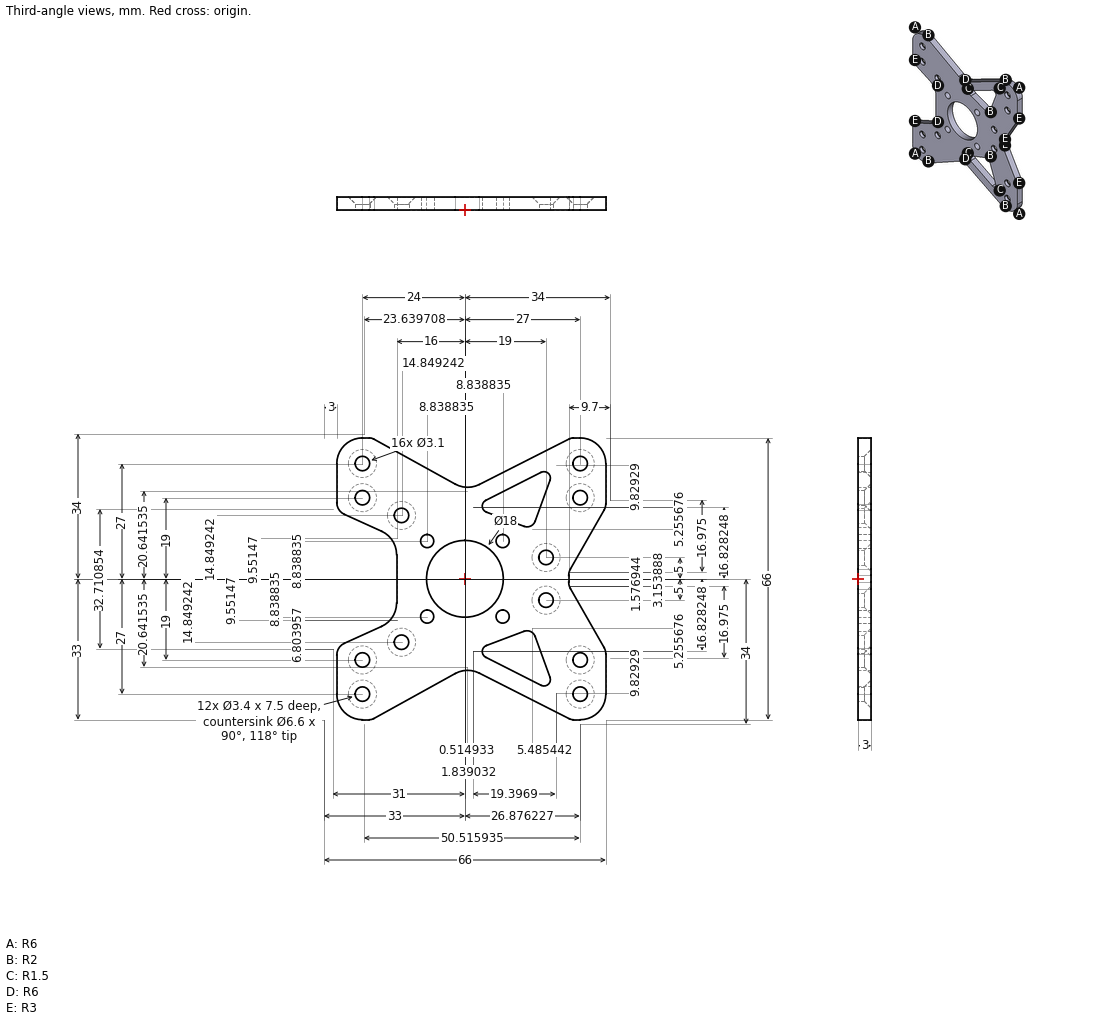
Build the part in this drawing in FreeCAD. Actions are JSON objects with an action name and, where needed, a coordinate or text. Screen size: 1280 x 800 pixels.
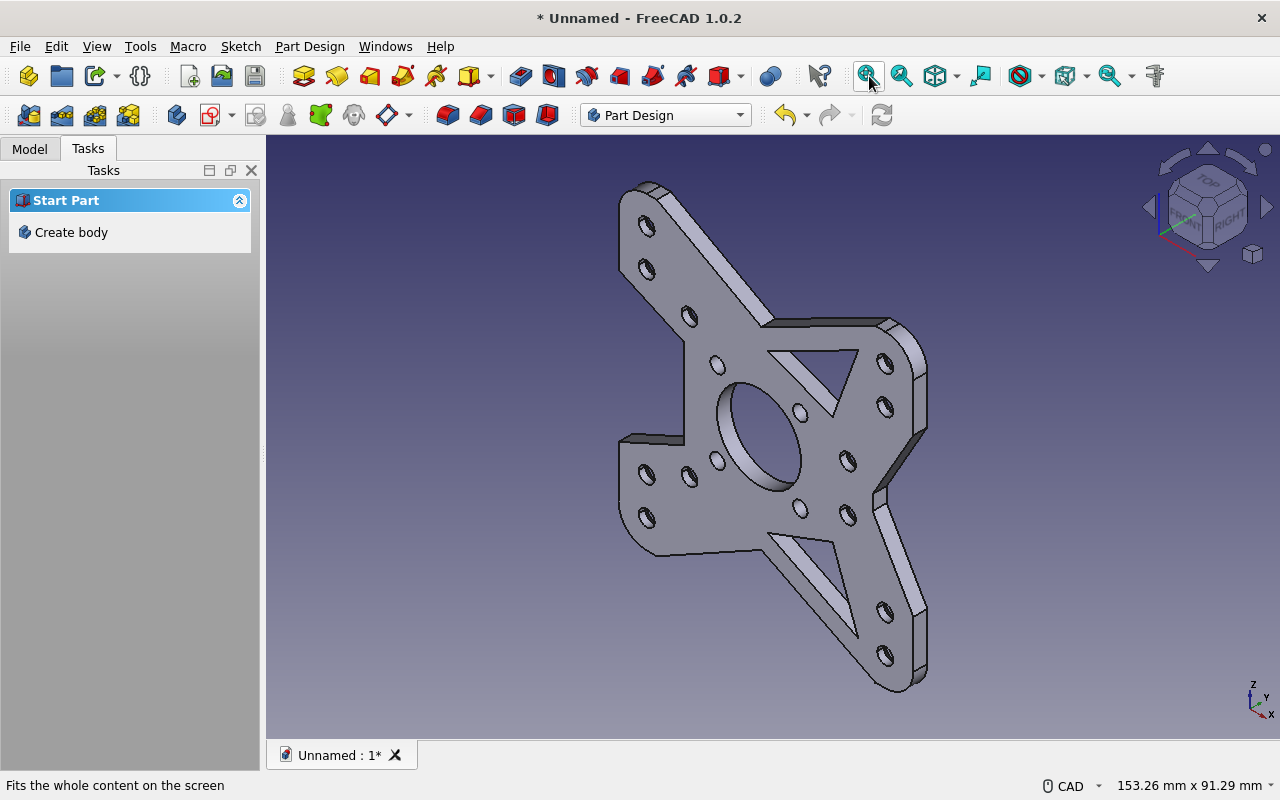
{"action": "key", "text": "2"}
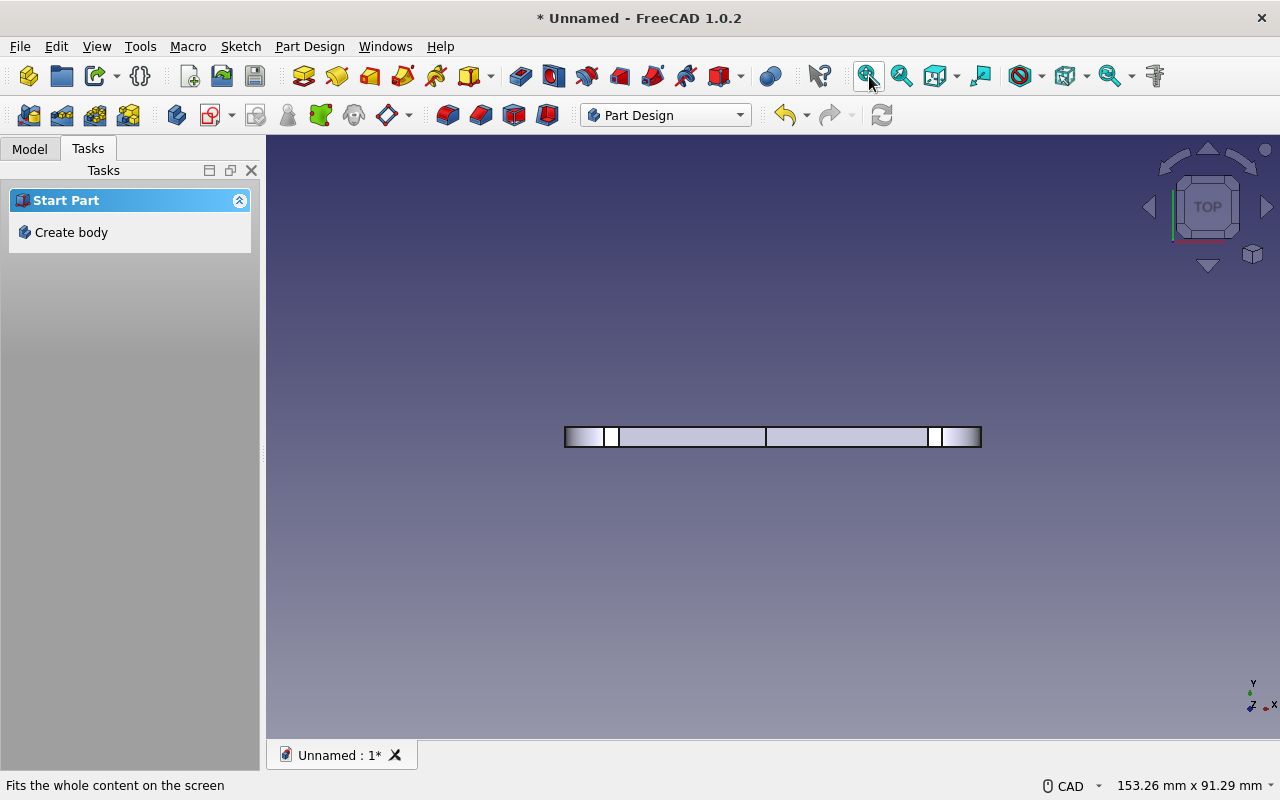
{"action": "key", "text": "v f"}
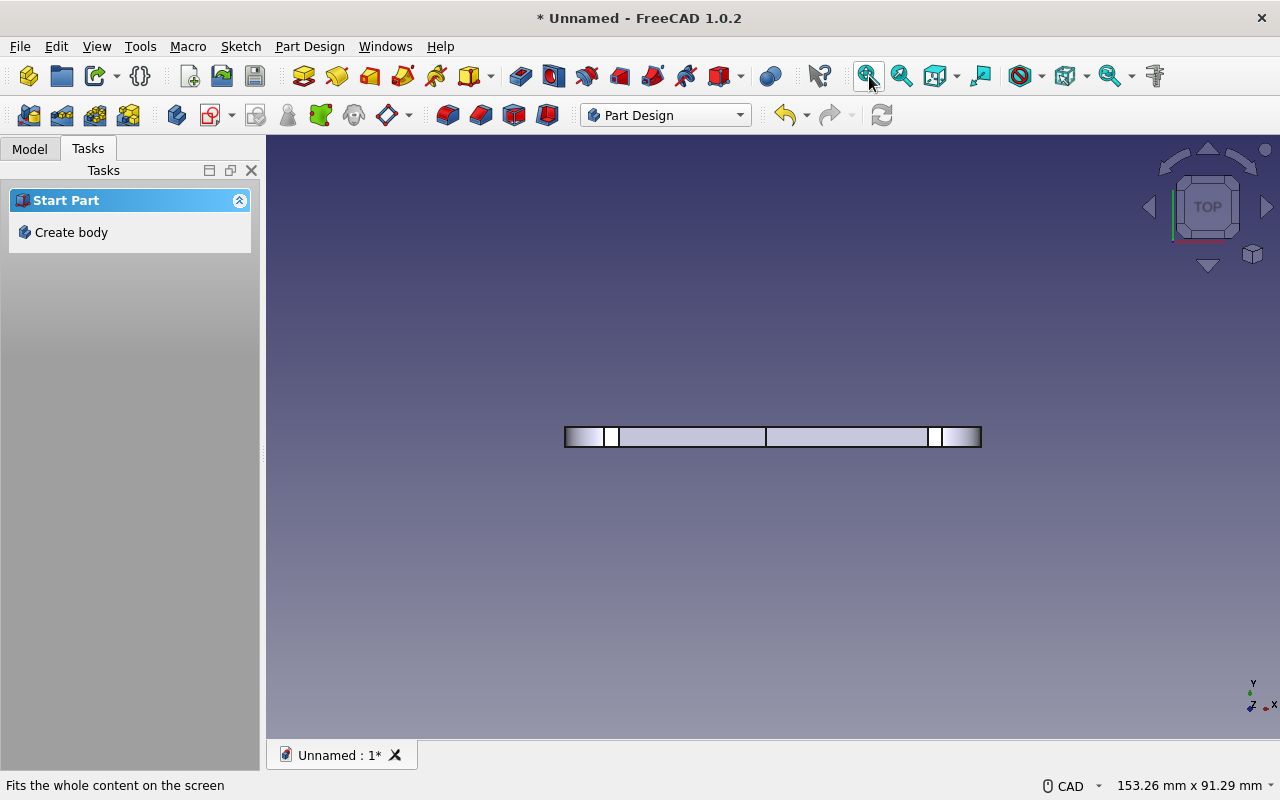
{"action": "left_click", "coordinate": [928, 436]}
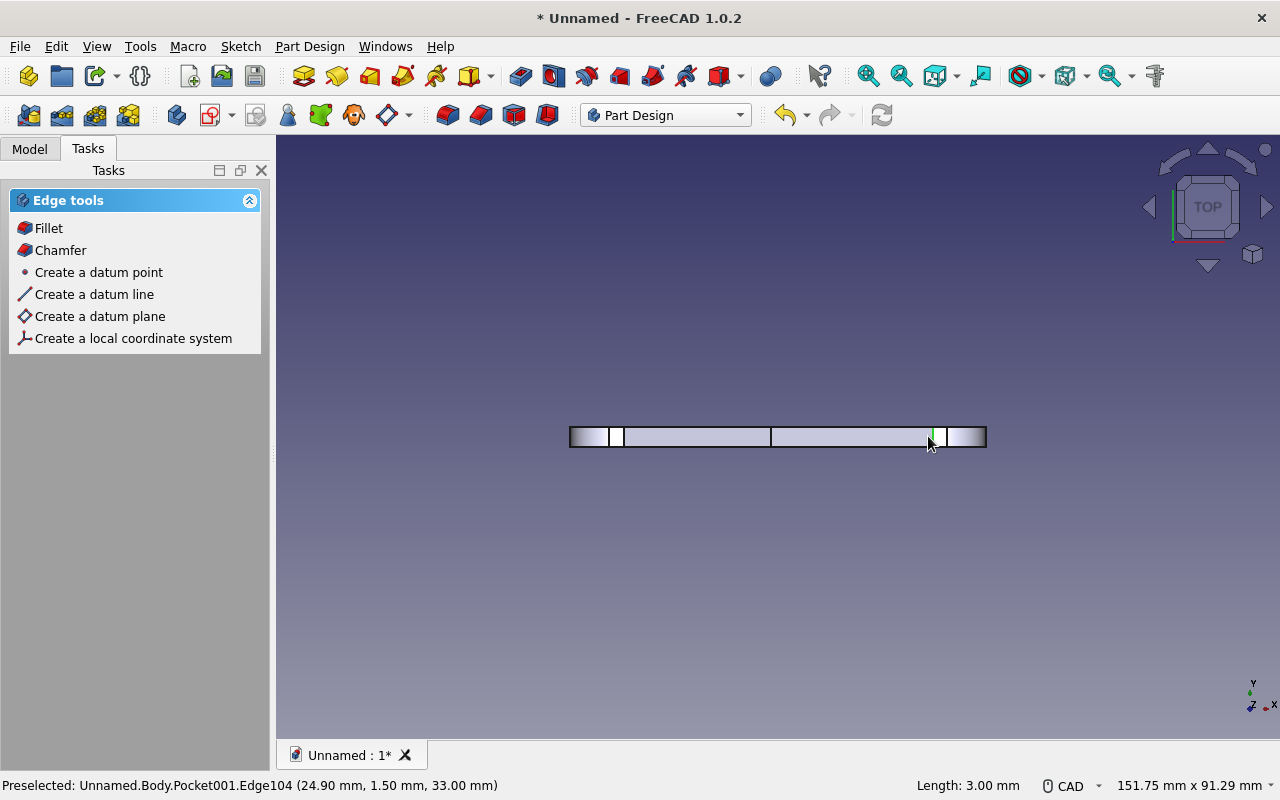
{"action": "left_click", "coordinate": [624, 436], "text": "ctrl"}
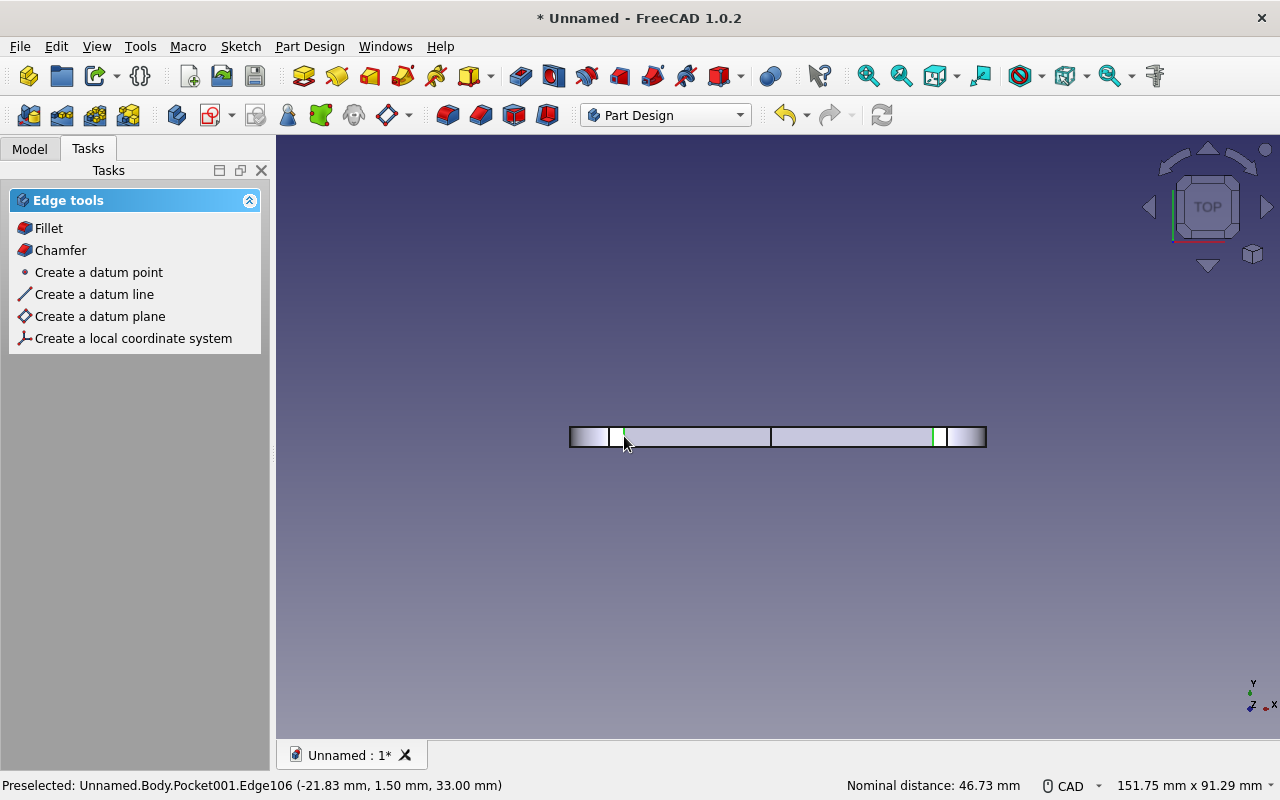
{"action": "scroll", "coordinate": [624, 436], "scroll_direction": "up", "scroll_amount": 4}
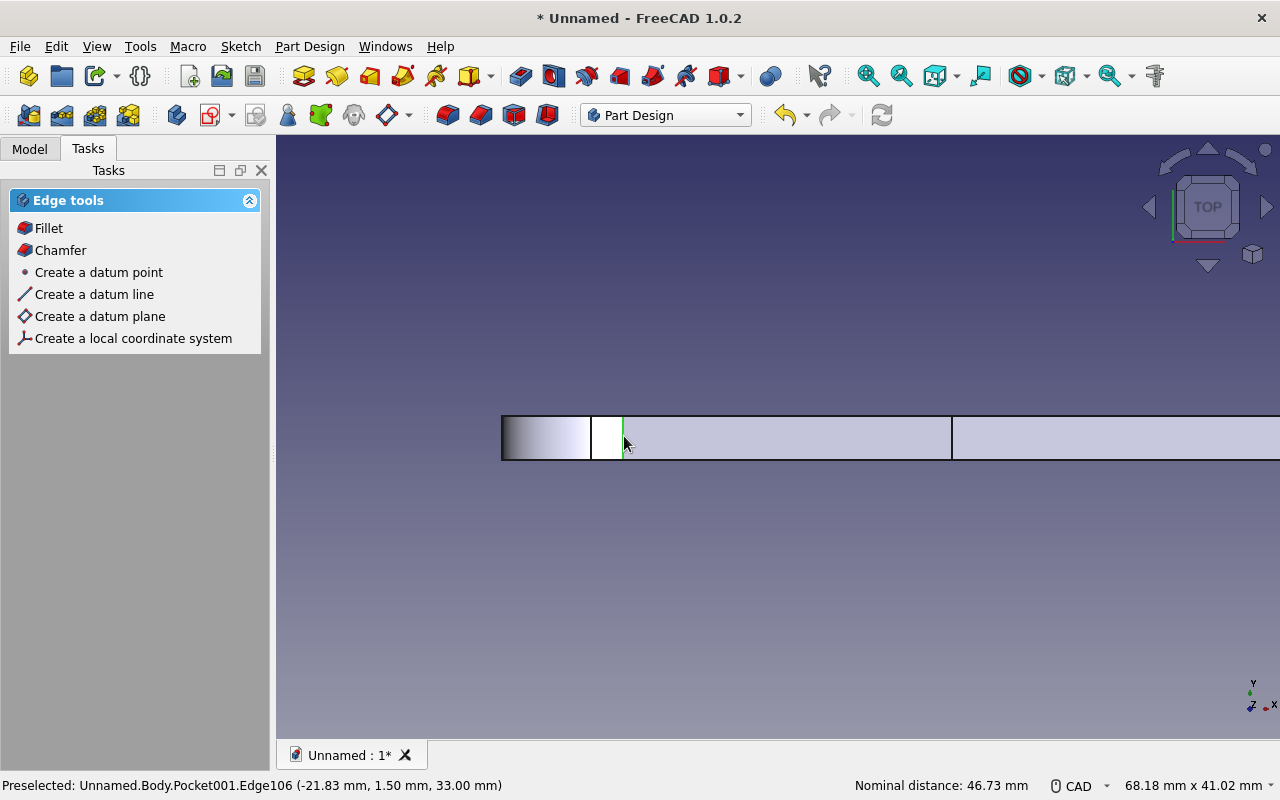
{"action": "left_click", "coordinate": [869, 76]}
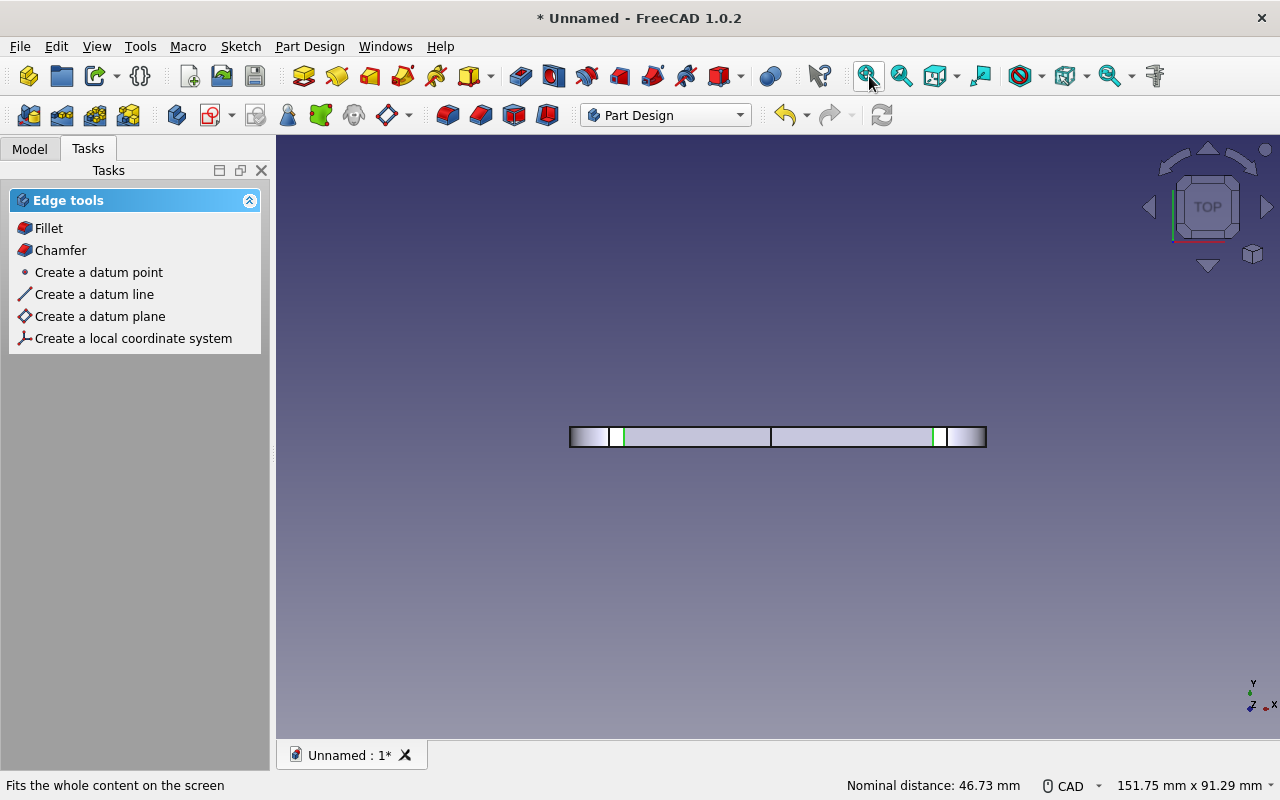
{"action": "key", "text": "1"}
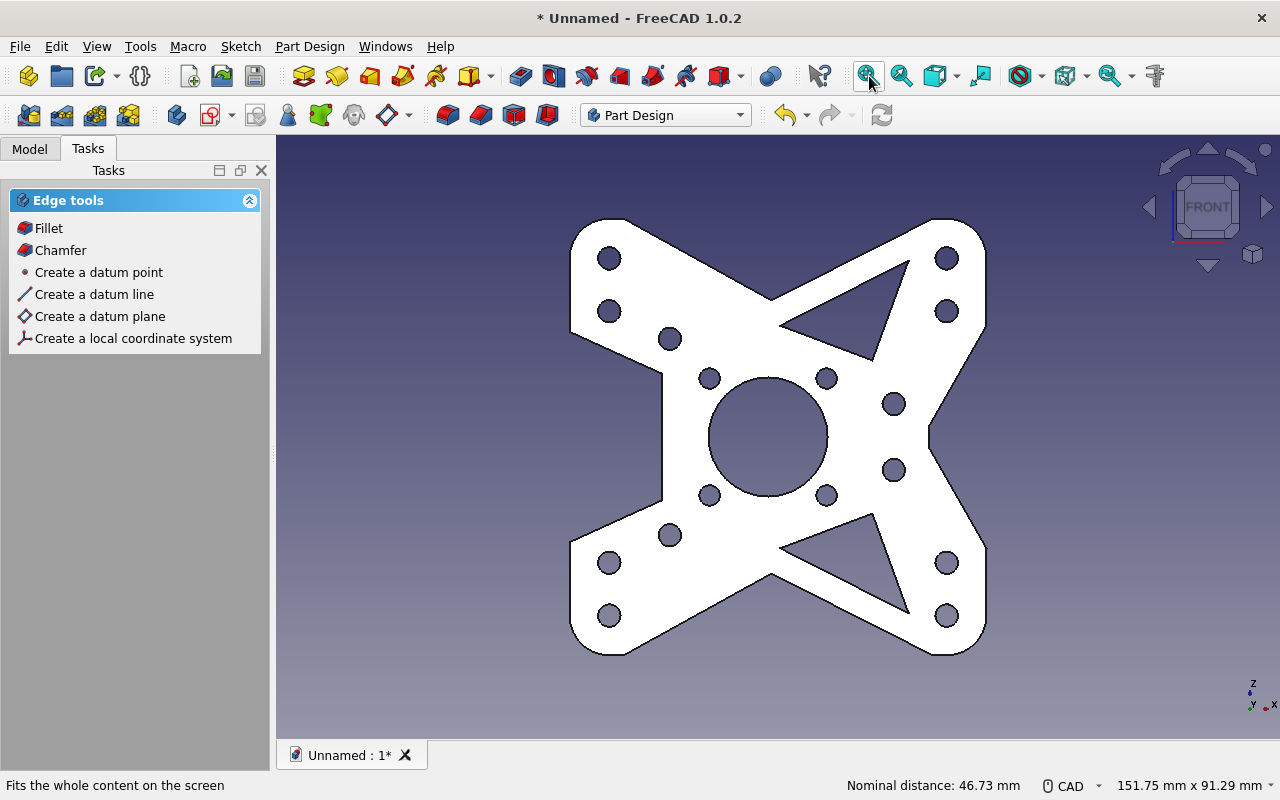
{"action": "scroll", "coordinate": [624, 654], "scroll_direction": "up", "scroll_amount": 4}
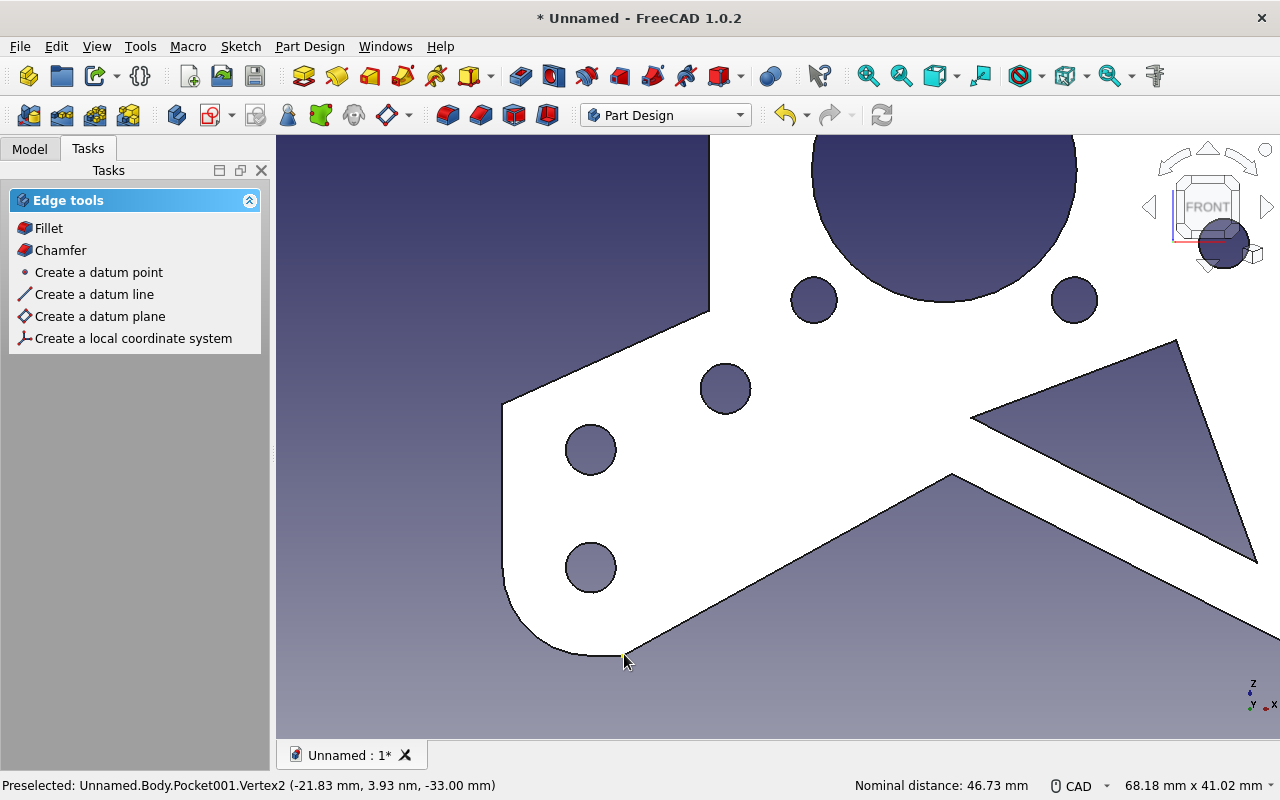
{"action": "key", "text": "v f"}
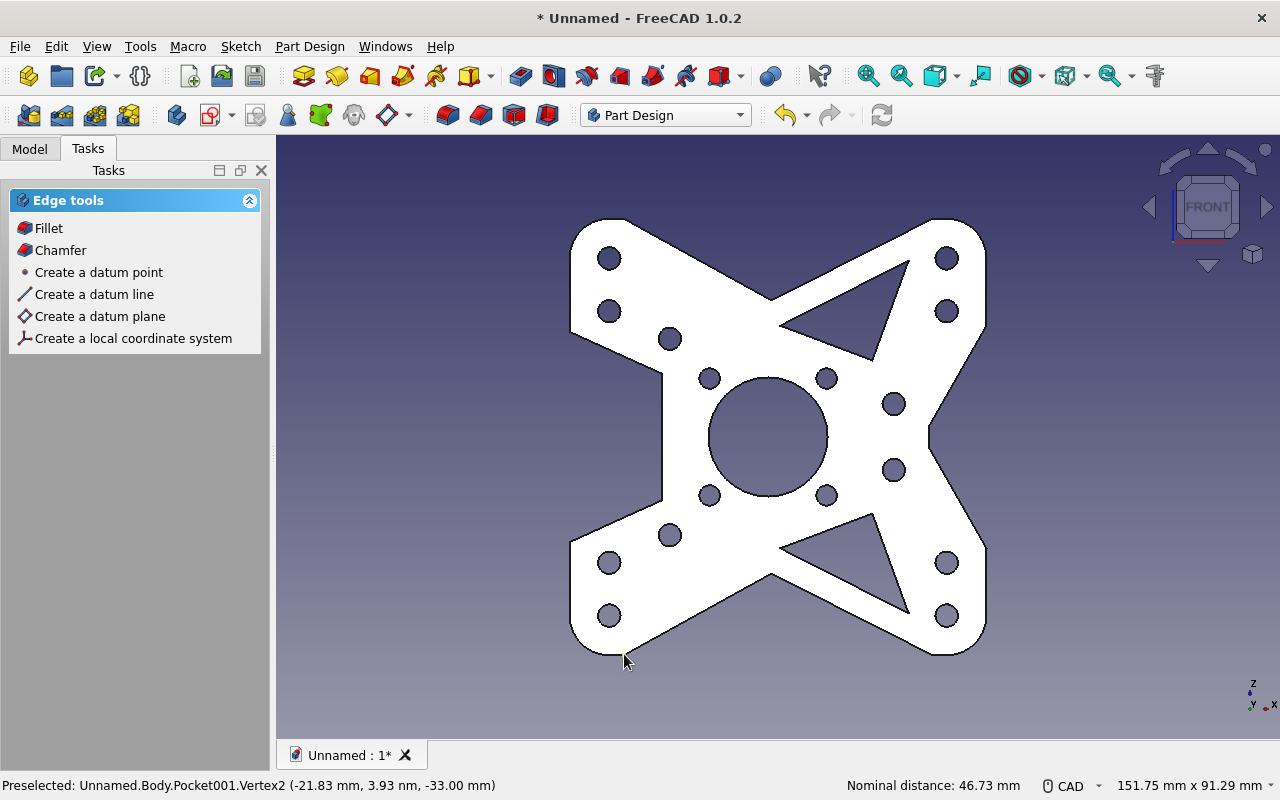
{"action": "key", "text": "3"}